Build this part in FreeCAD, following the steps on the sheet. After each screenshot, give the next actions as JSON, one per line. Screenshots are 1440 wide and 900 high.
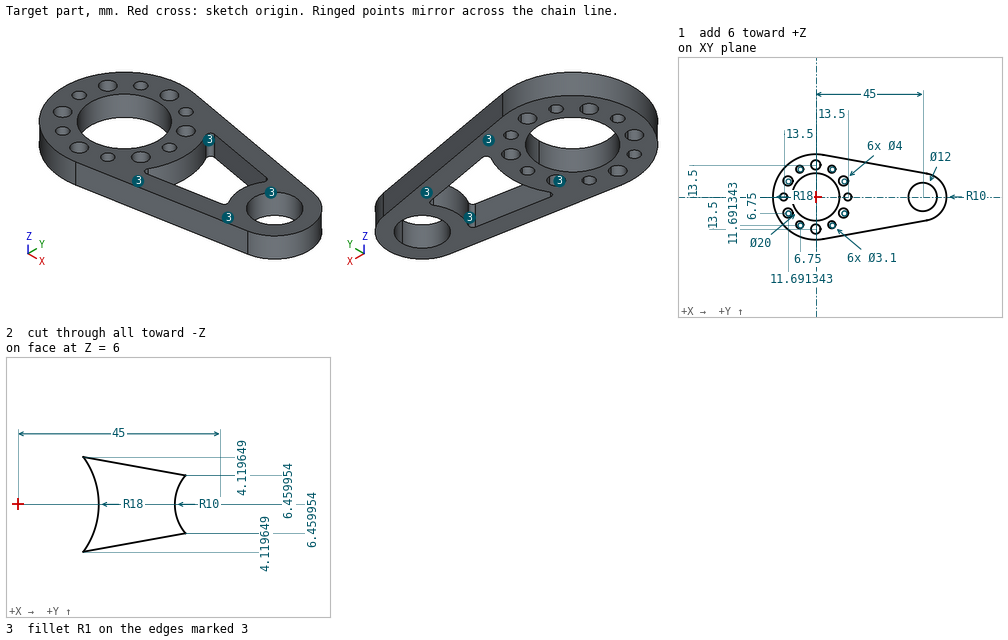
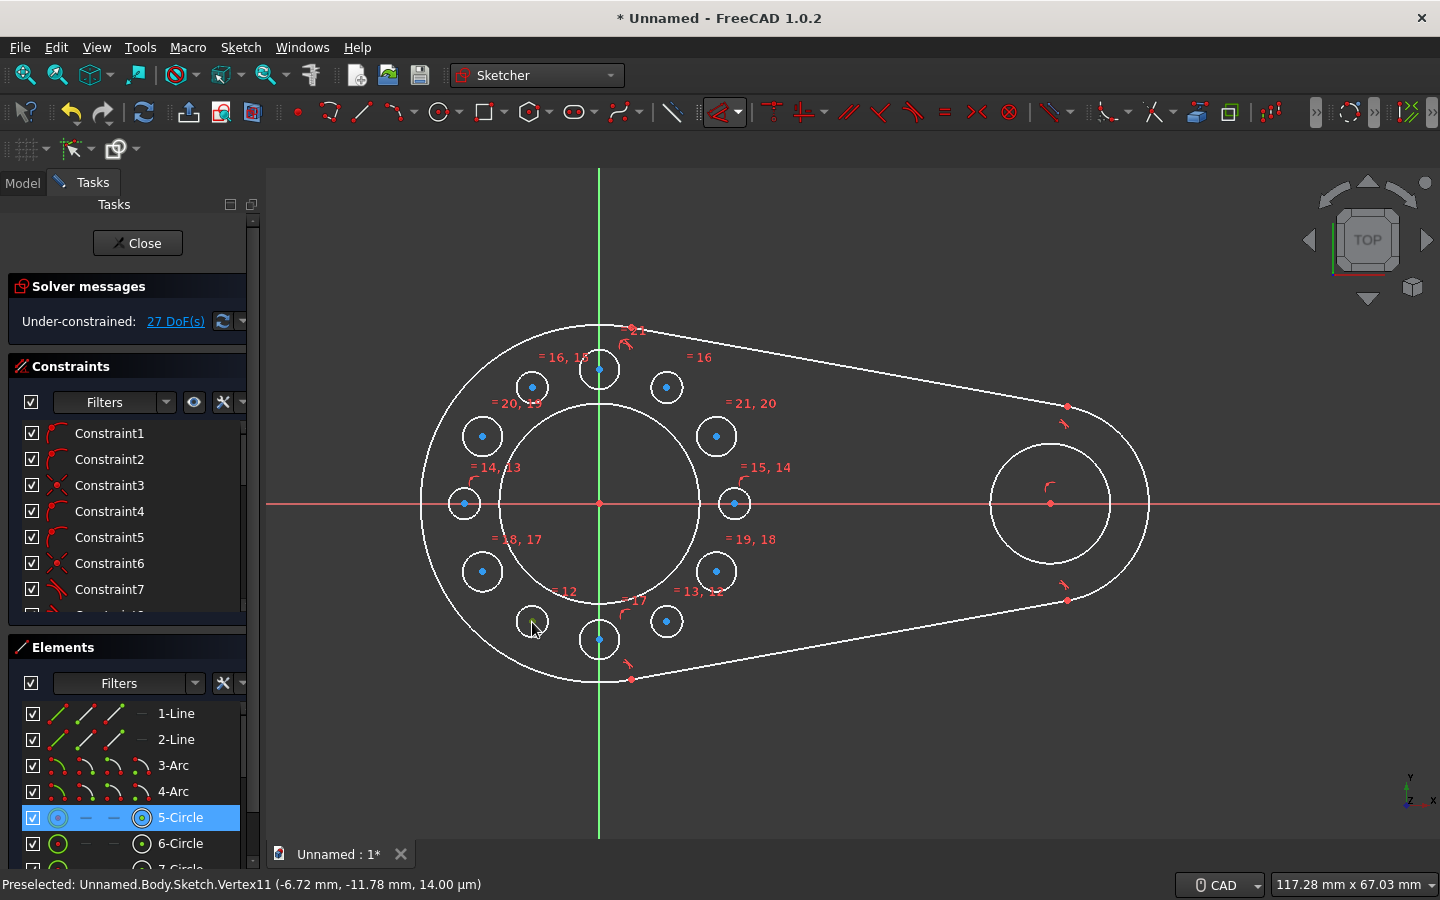
{"action": "left_click", "coordinate": [667, 622]}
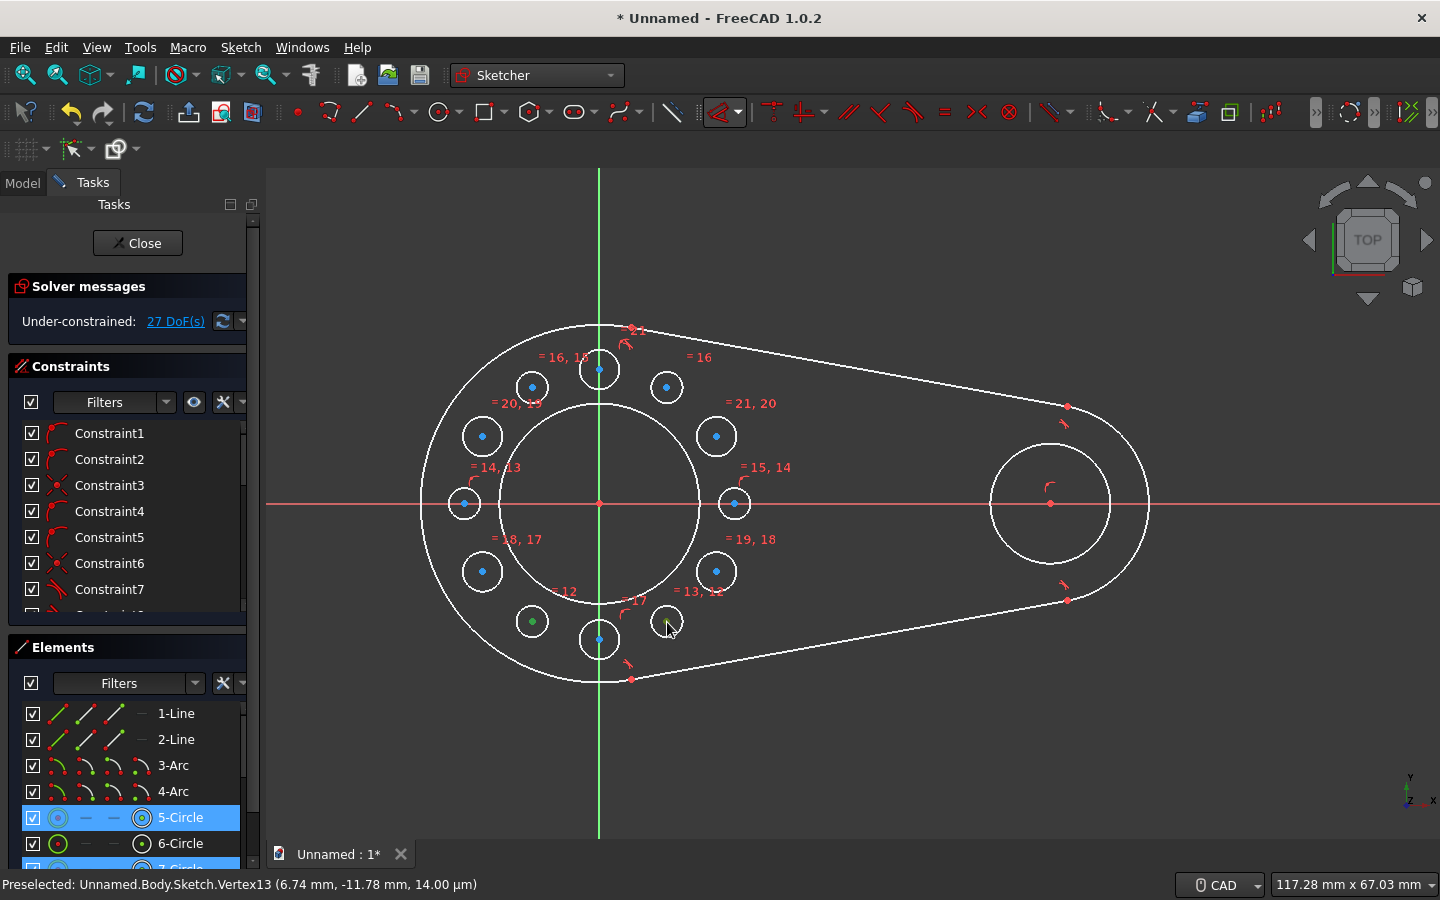
{"action": "left_click", "coordinate": [599, 767]}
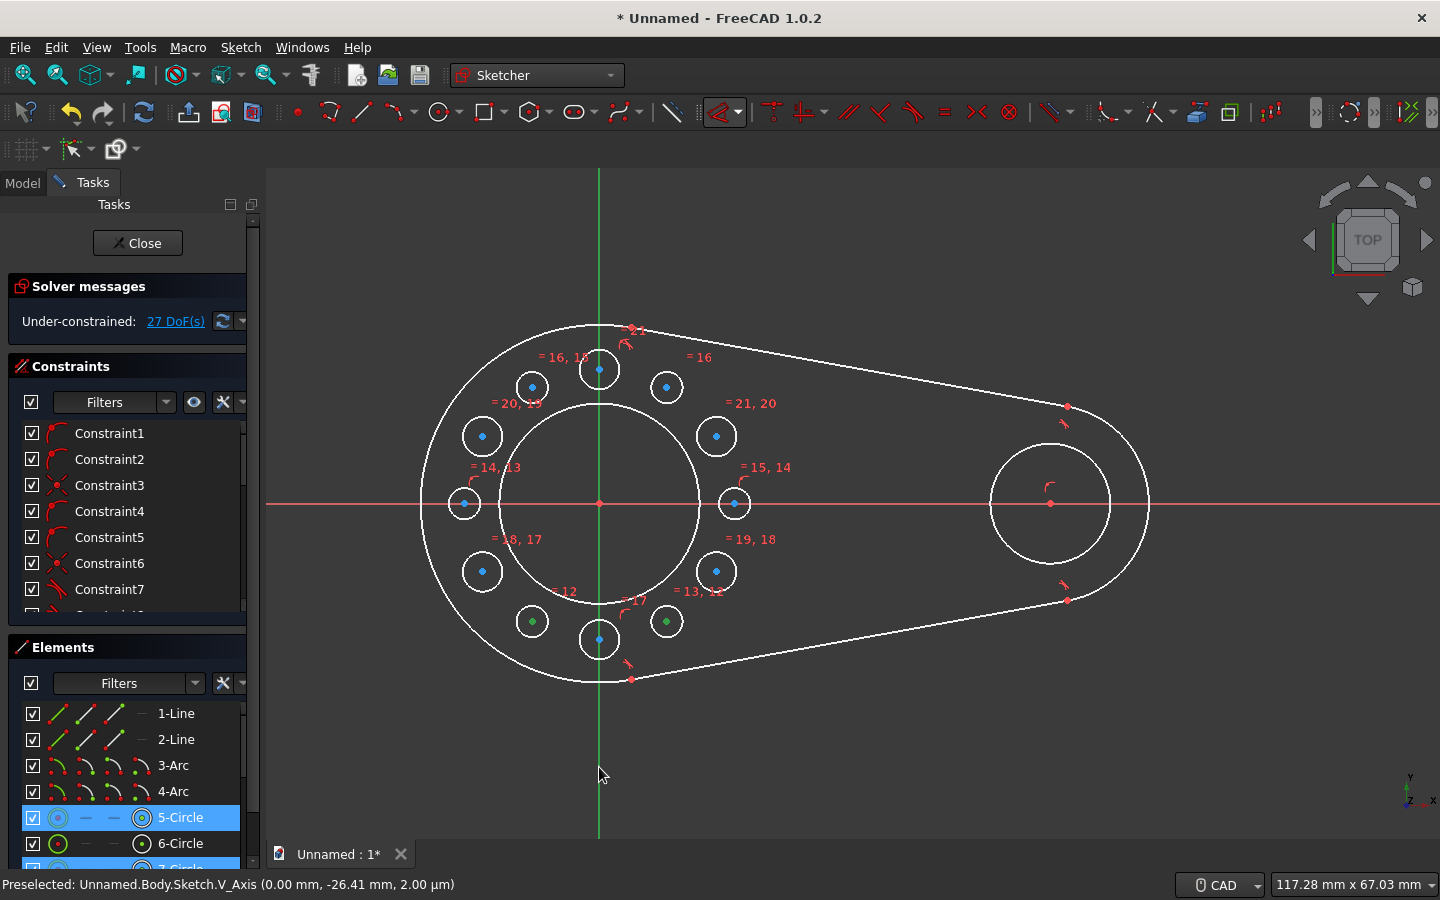
{"action": "key", "text": "s"}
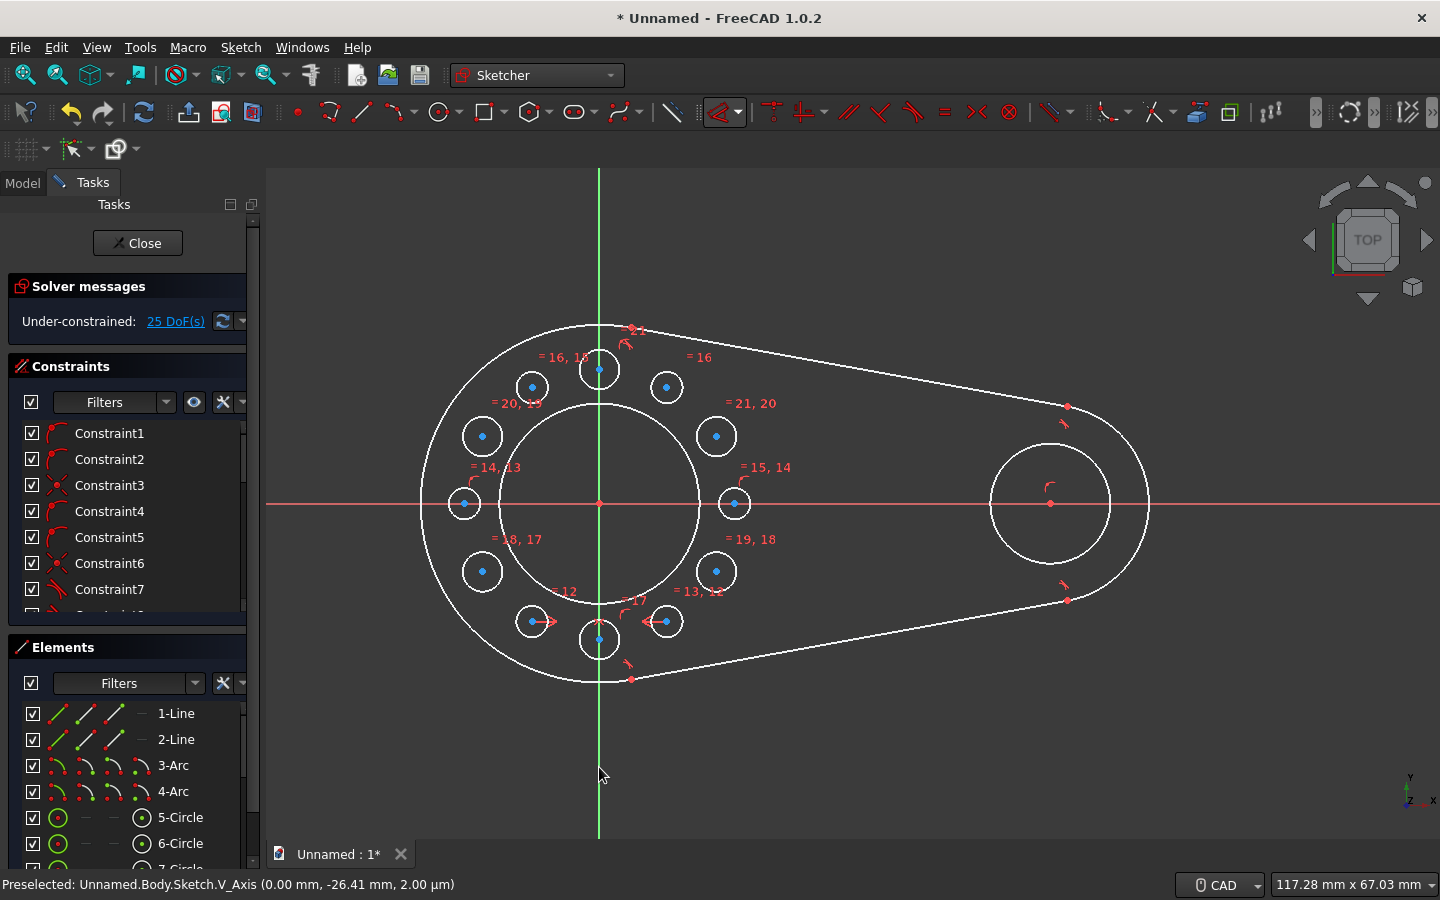
{"action": "left_click", "coordinate": [483, 572]}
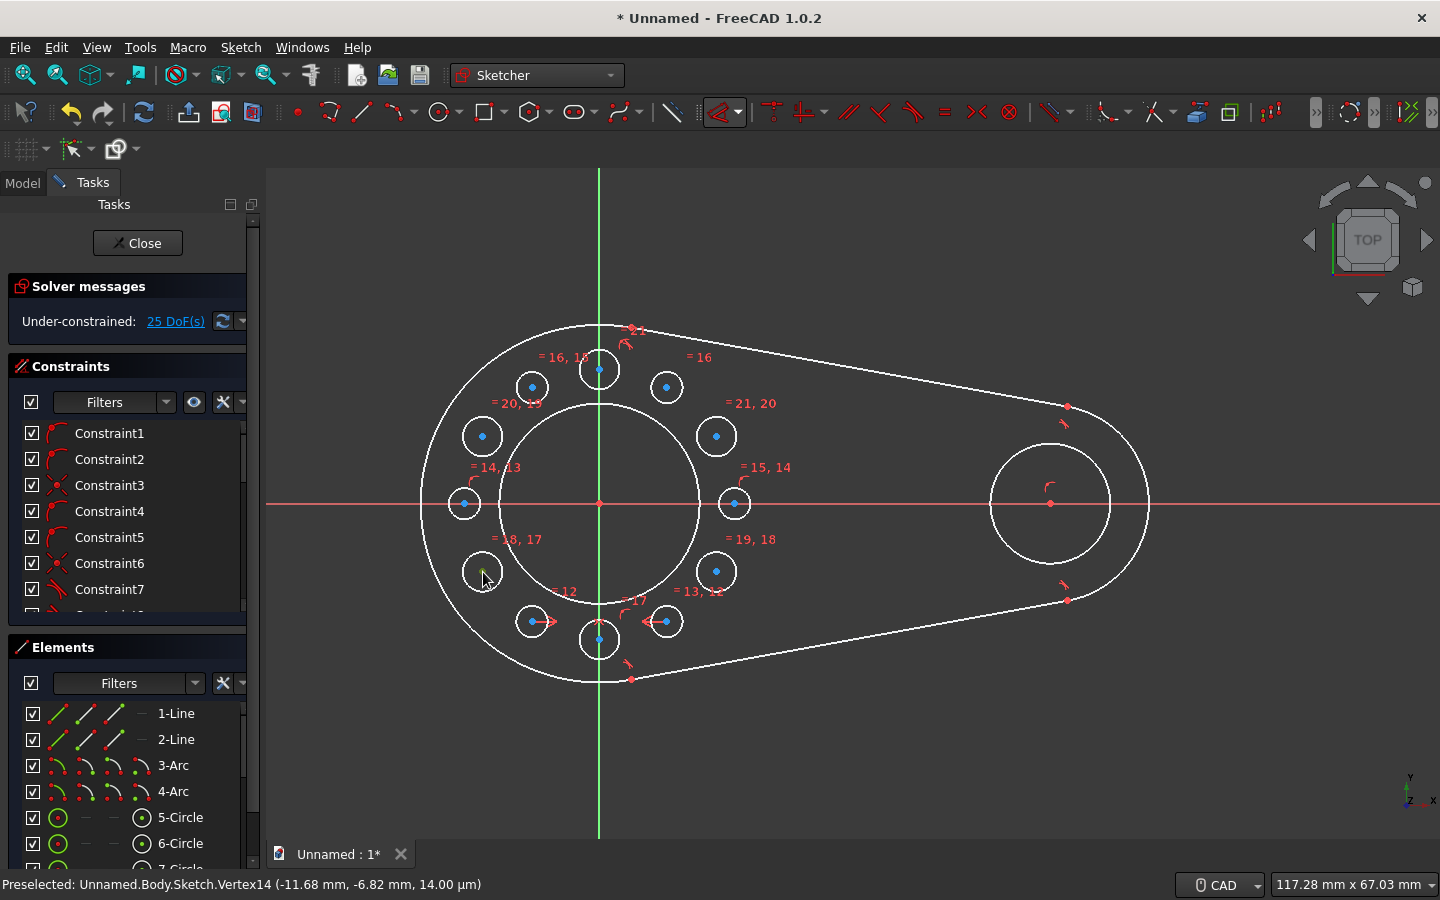
{"action": "left_click", "coordinate": [717, 572]}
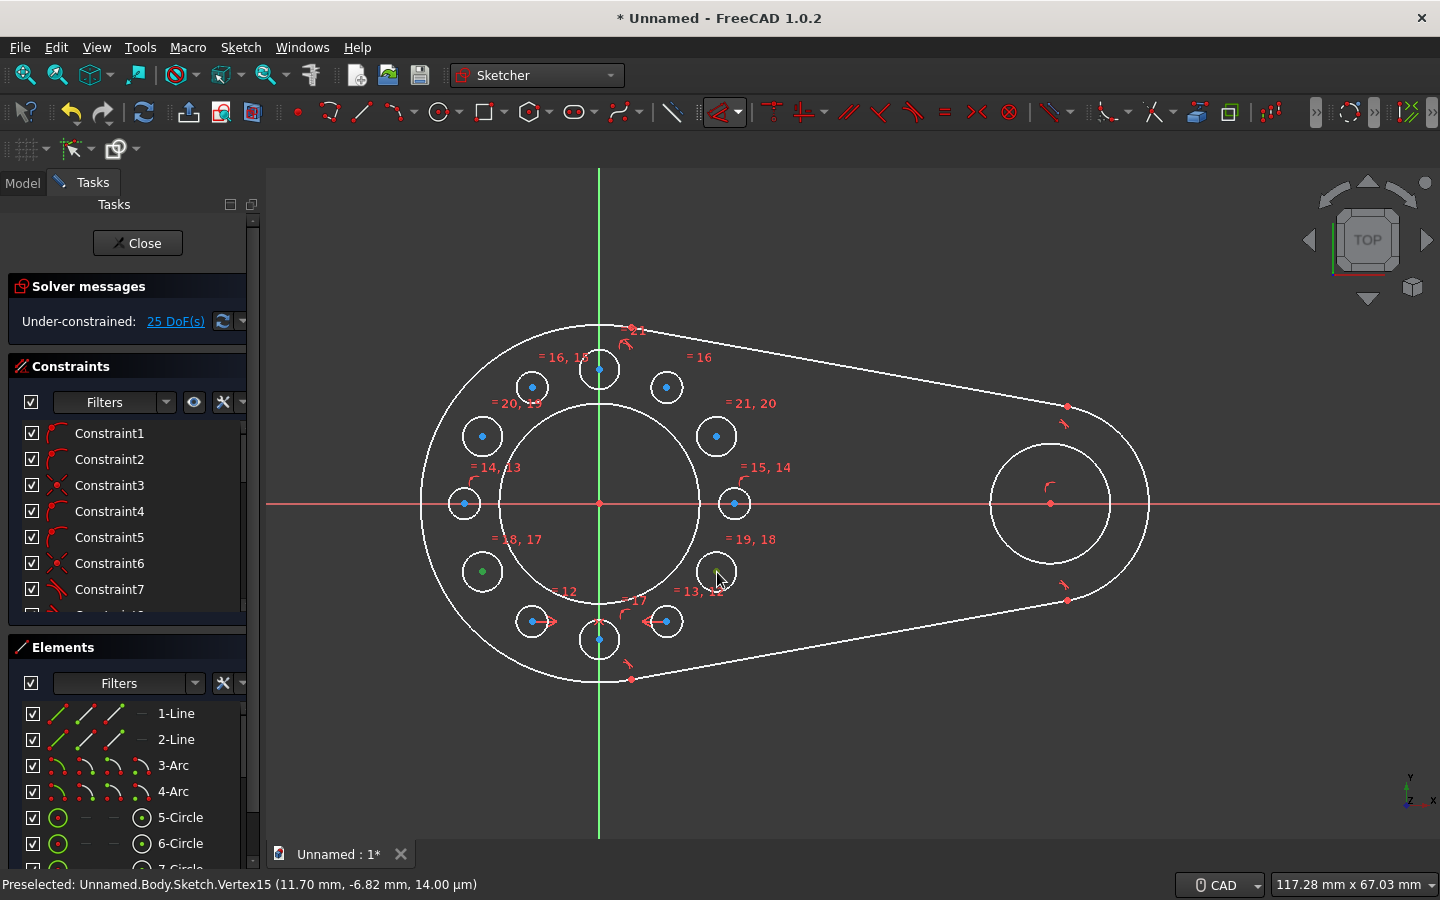
{"action": "left_click", "coordinate": [599, 767]}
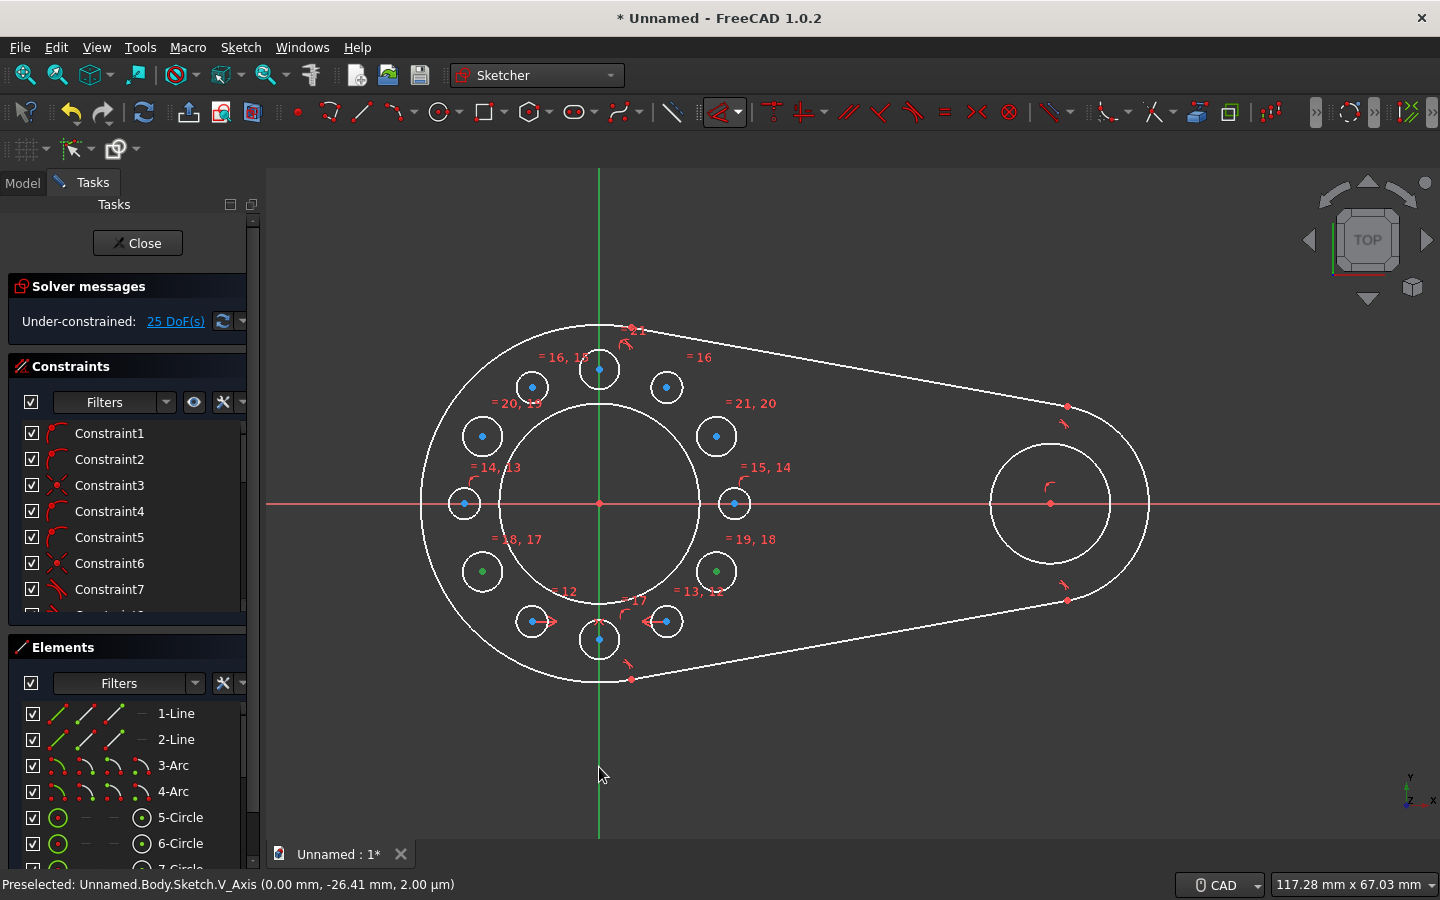
{"action": "key", "text": "s"}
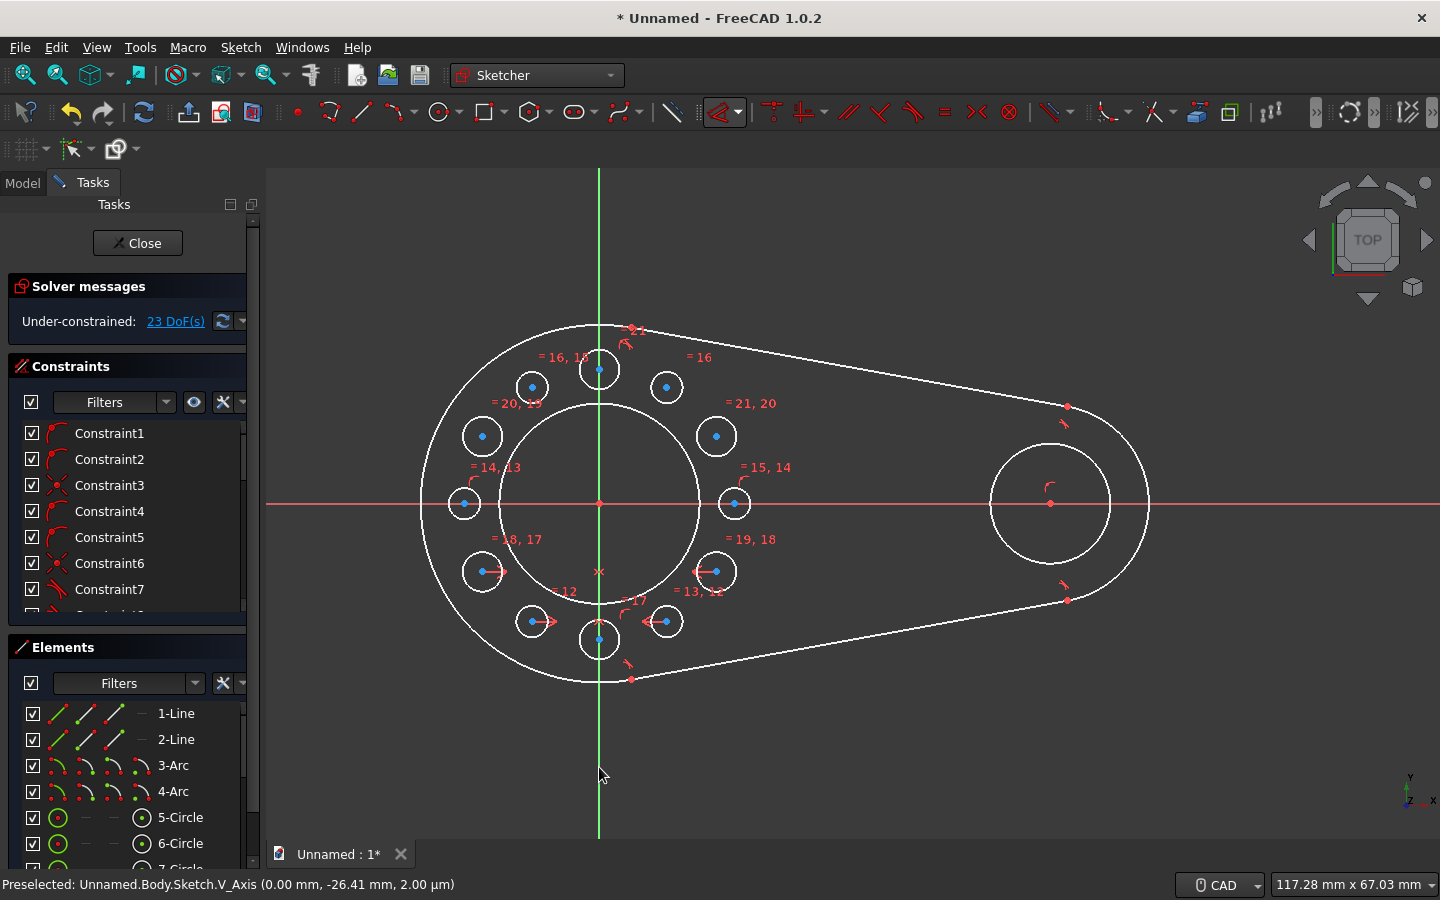
{"action": "left_click", "coordinate": [482, 572]}